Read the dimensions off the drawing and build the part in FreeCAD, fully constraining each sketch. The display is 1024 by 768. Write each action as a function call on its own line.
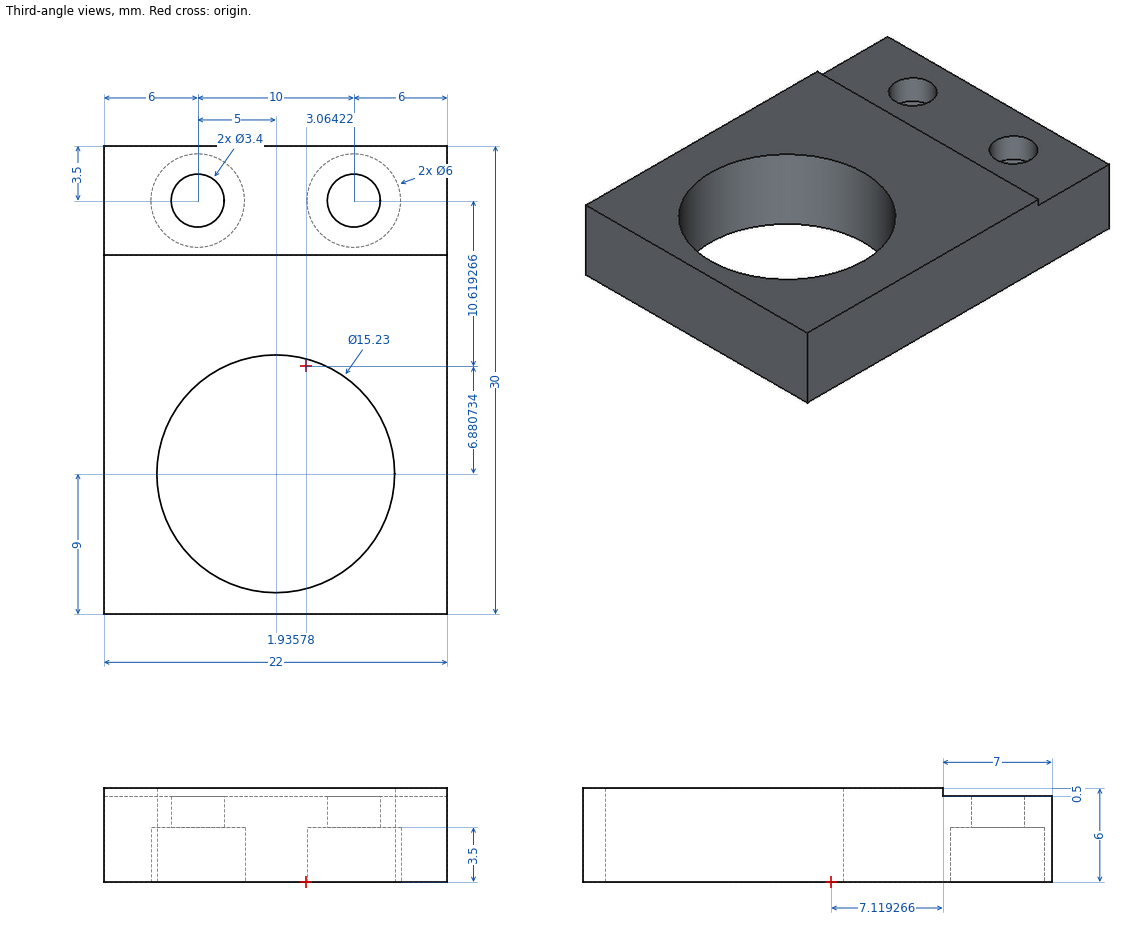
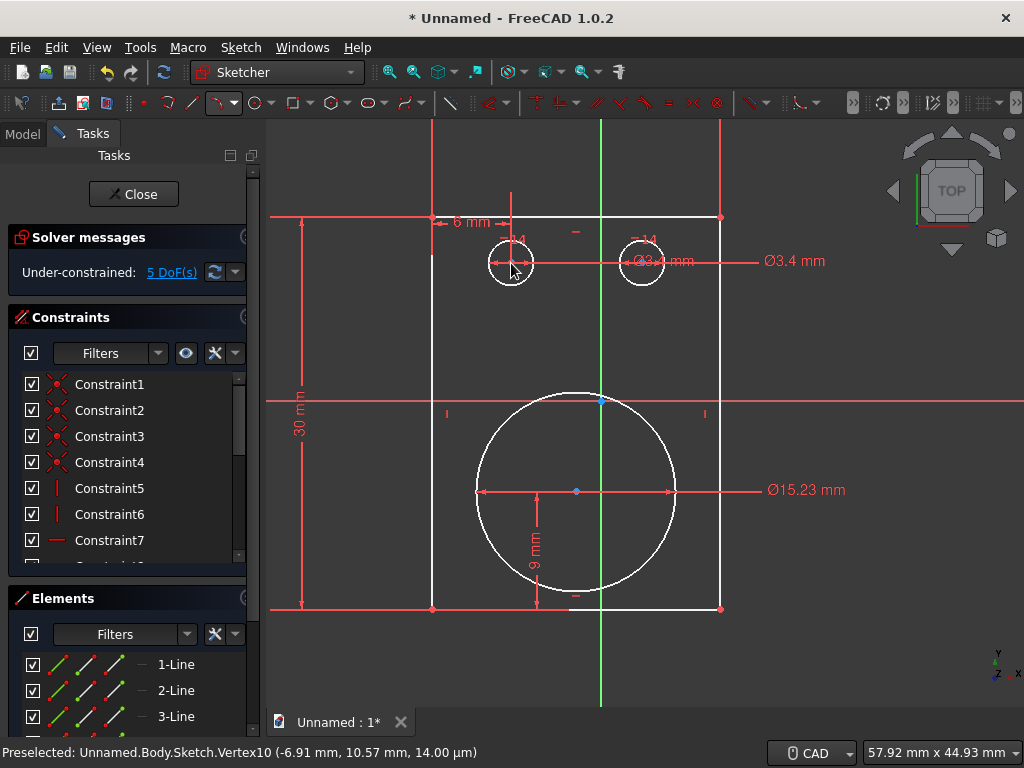
click(576, 492)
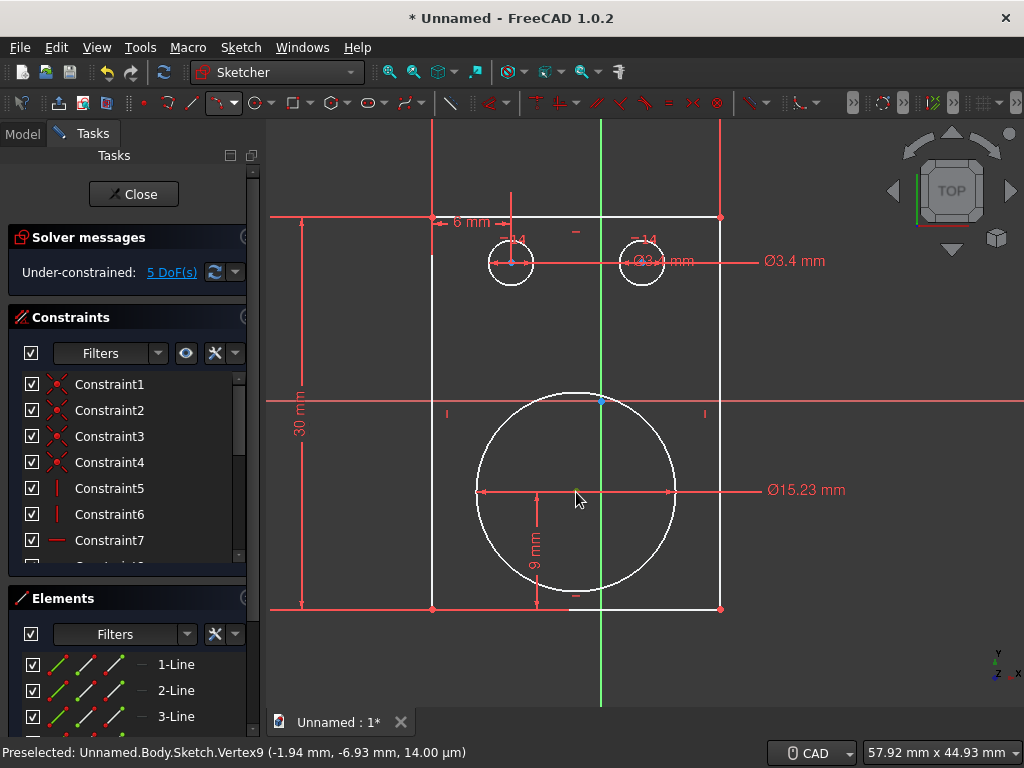
click(511, 263)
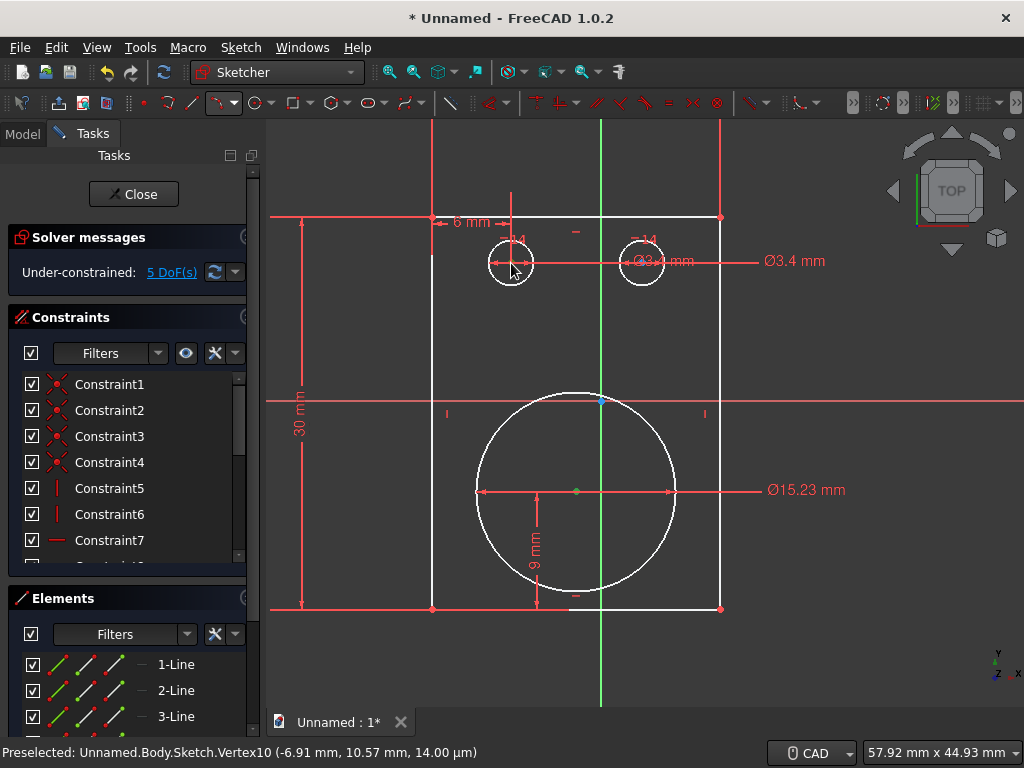
key(l)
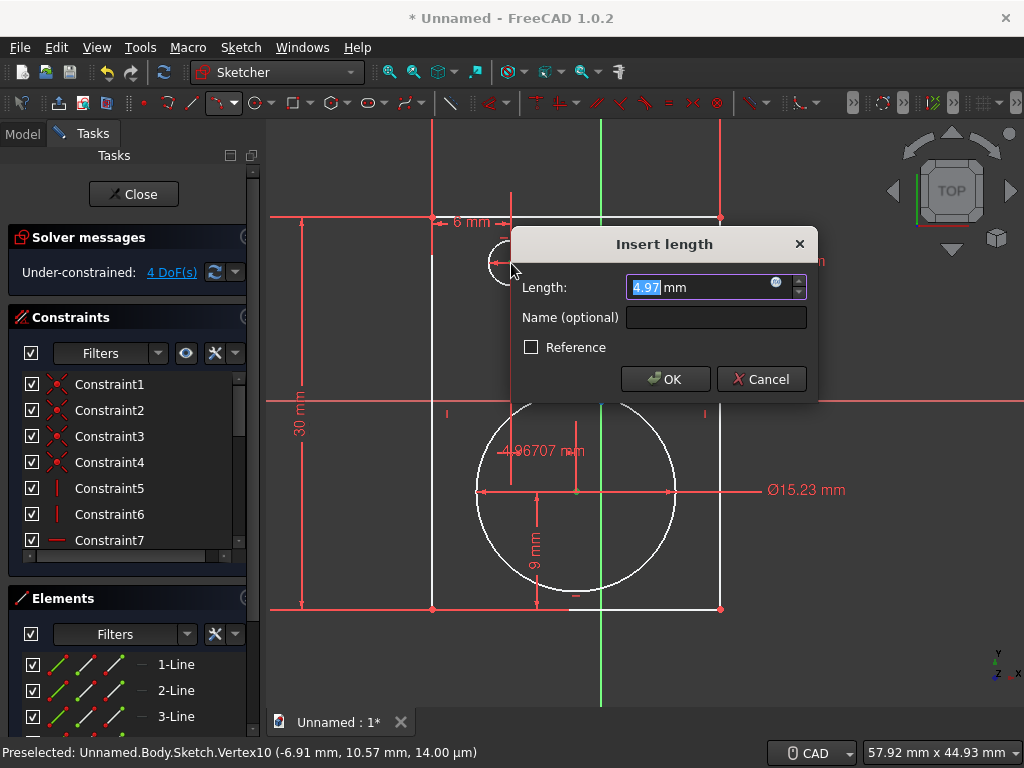
text(5)
key(Return)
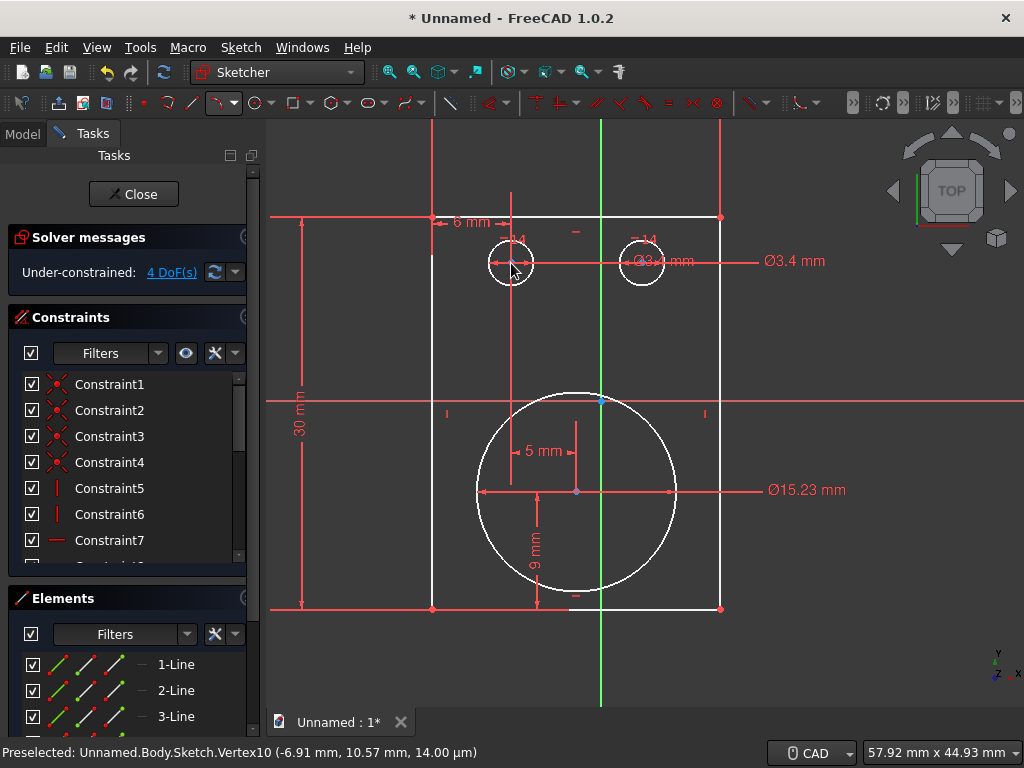
click(720, 217)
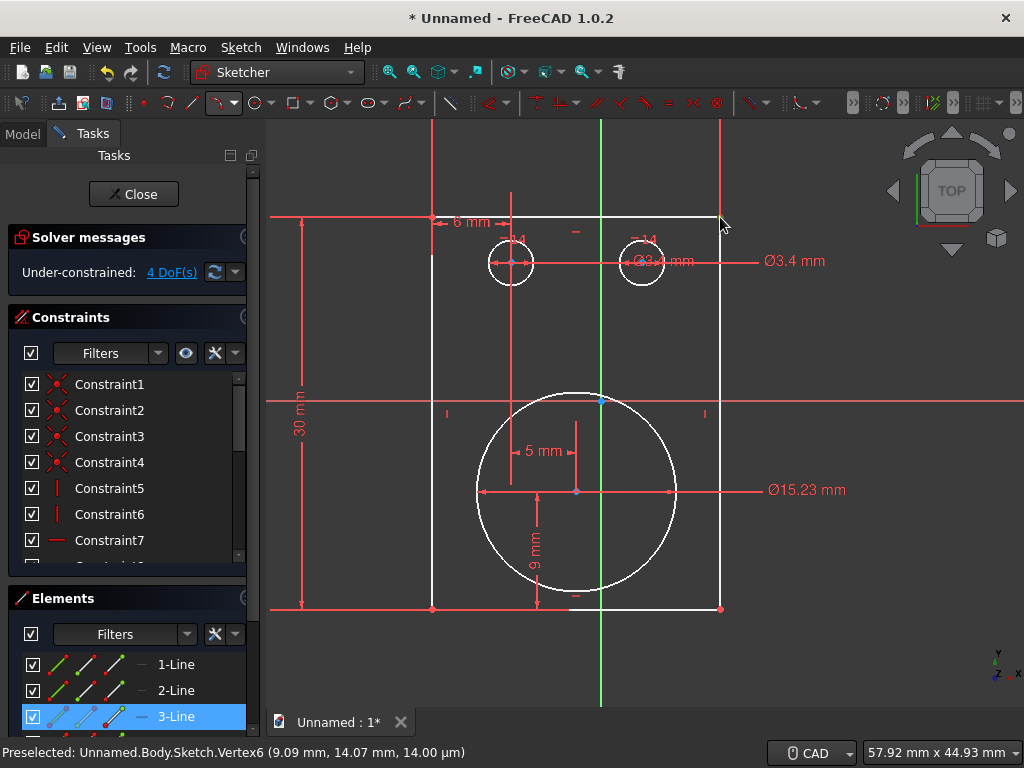
click(642, 263)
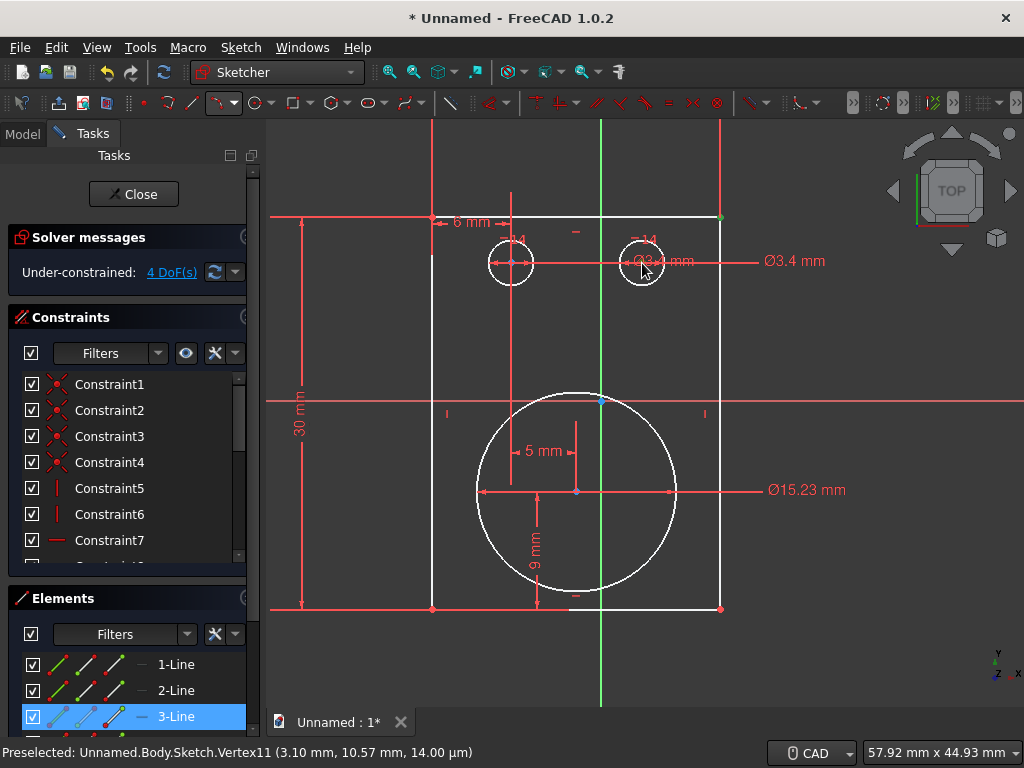
key(l)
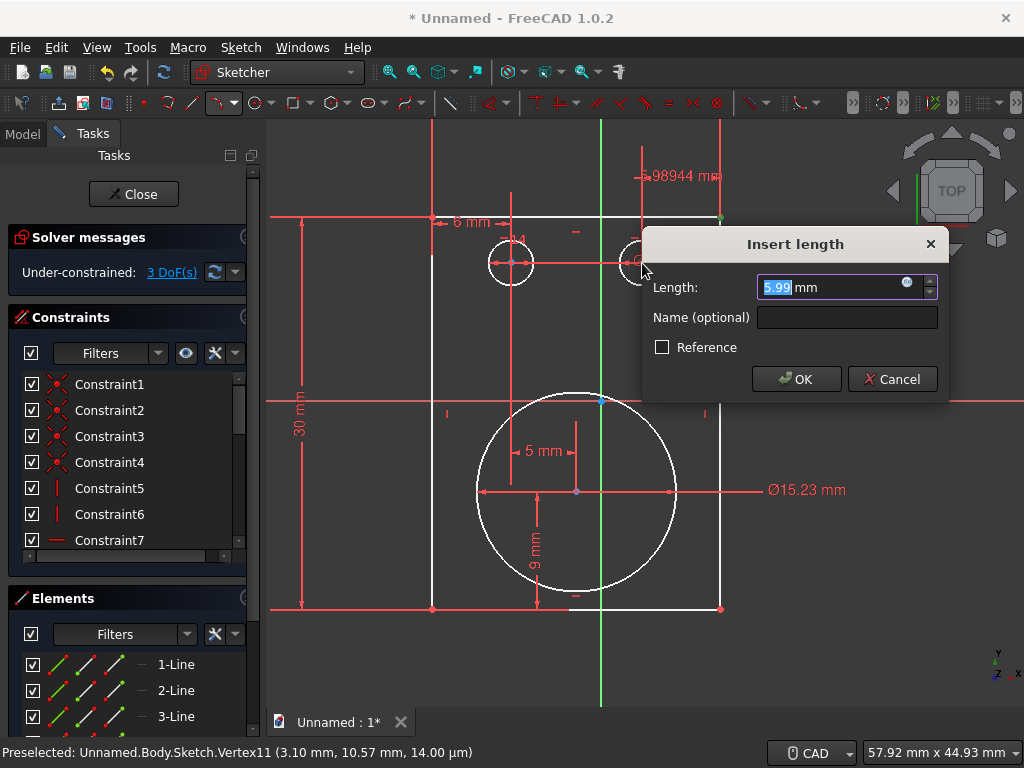
text(6)
key(Return)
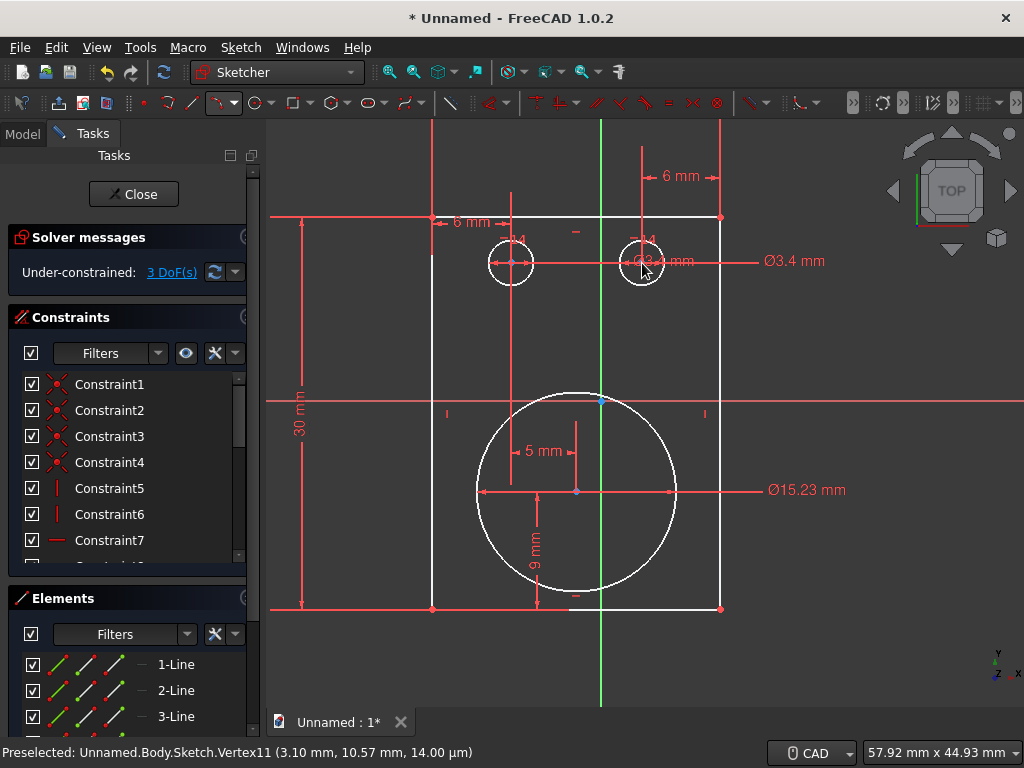
click(432, 217)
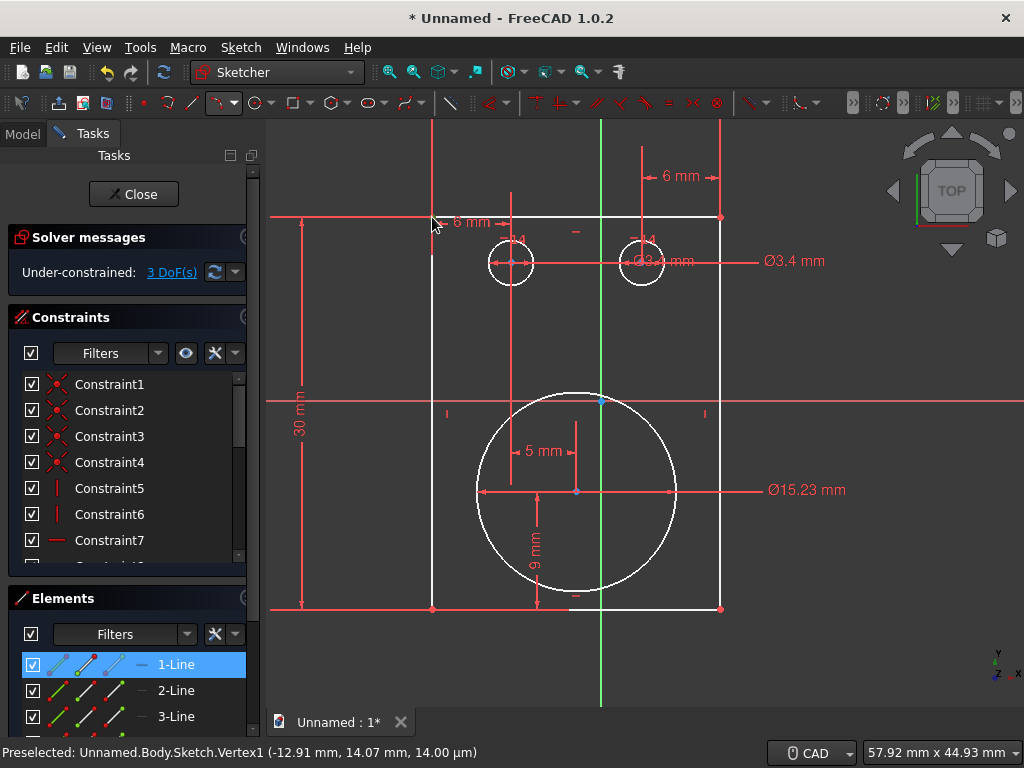
click(511, 263)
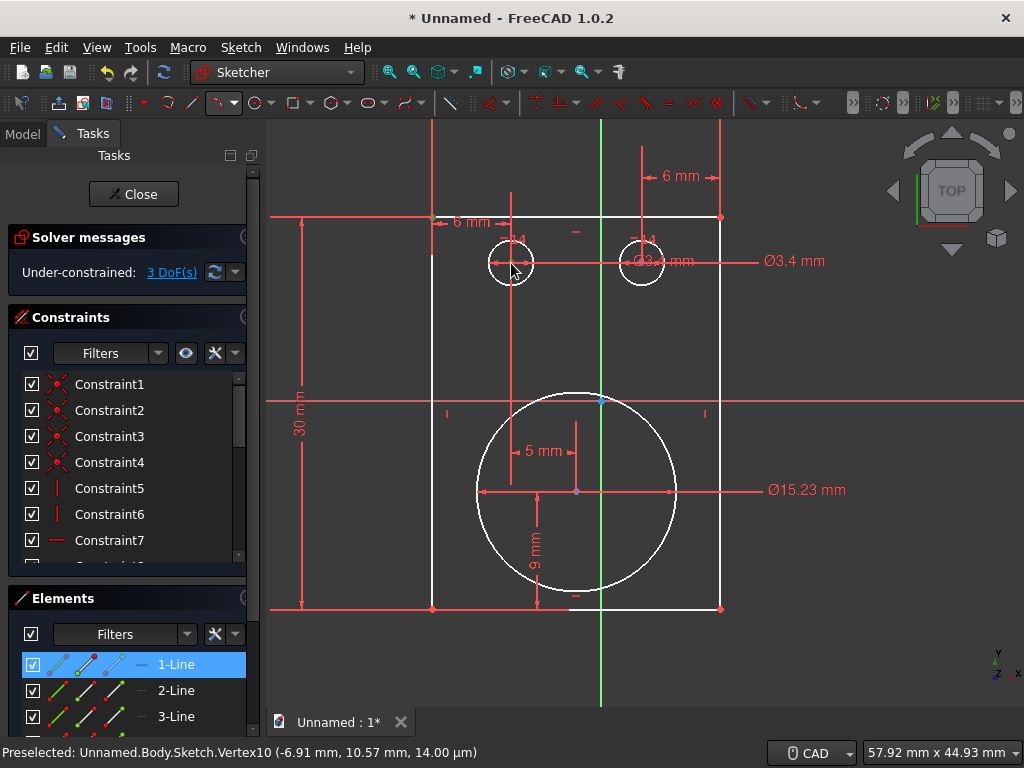
key(i)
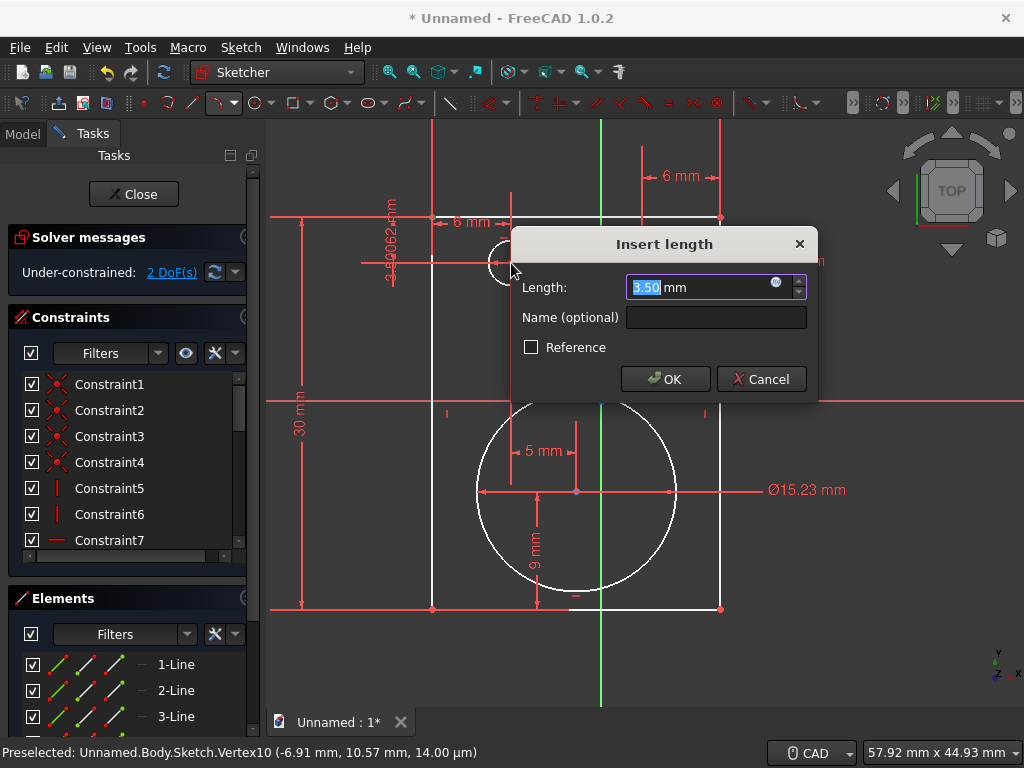
text(3.5)
key(Return)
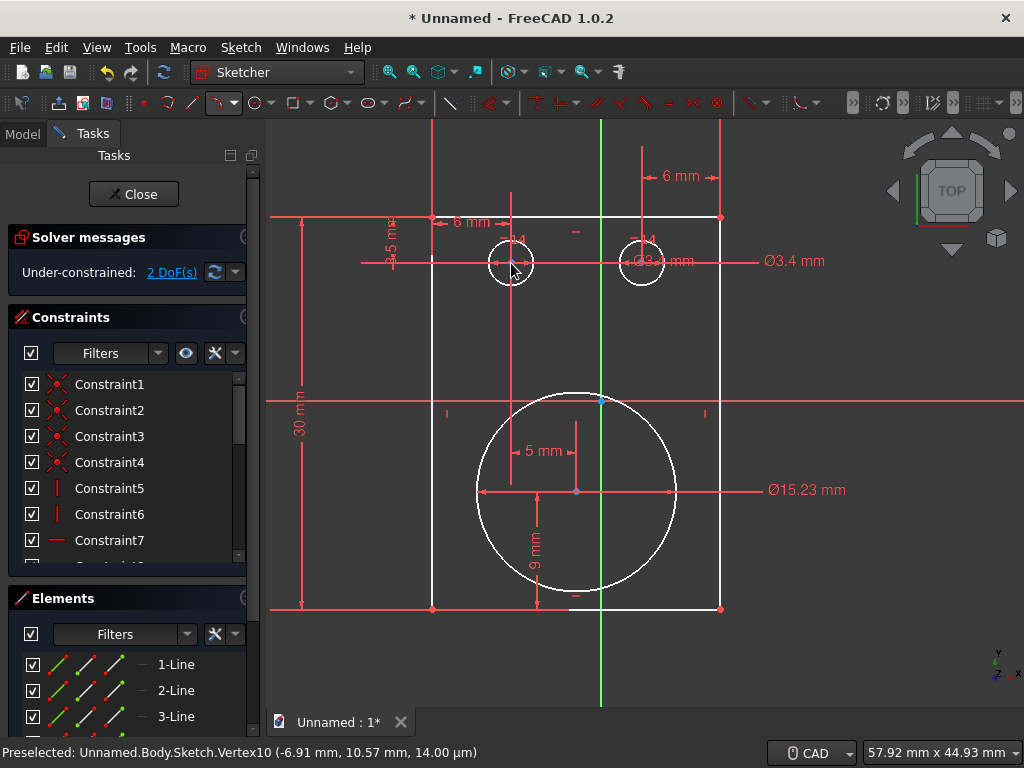
scroll(576, 492, up, 3)